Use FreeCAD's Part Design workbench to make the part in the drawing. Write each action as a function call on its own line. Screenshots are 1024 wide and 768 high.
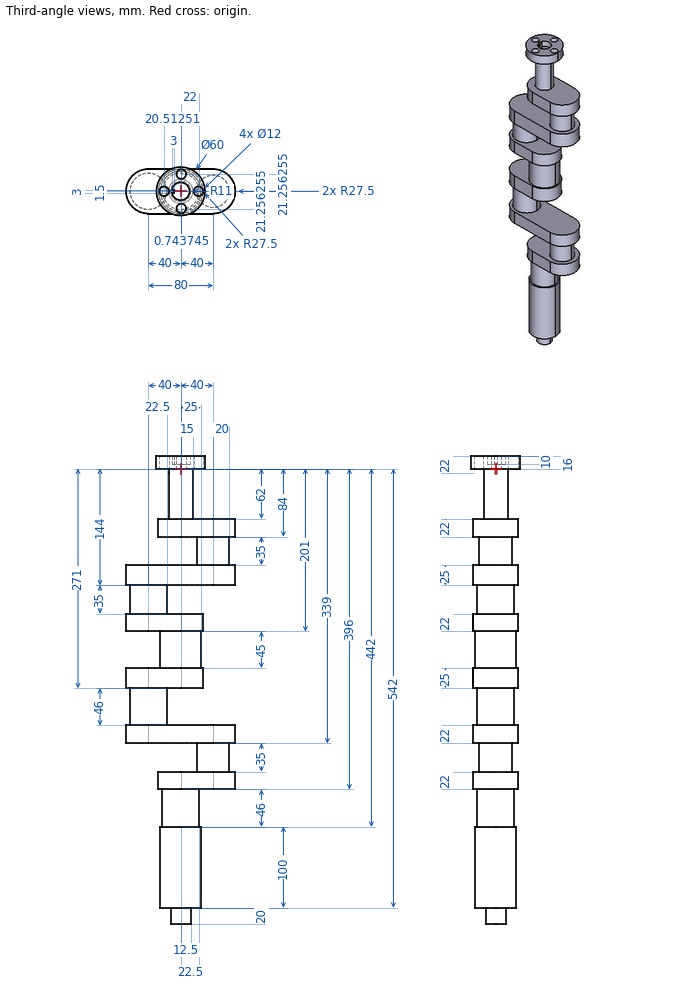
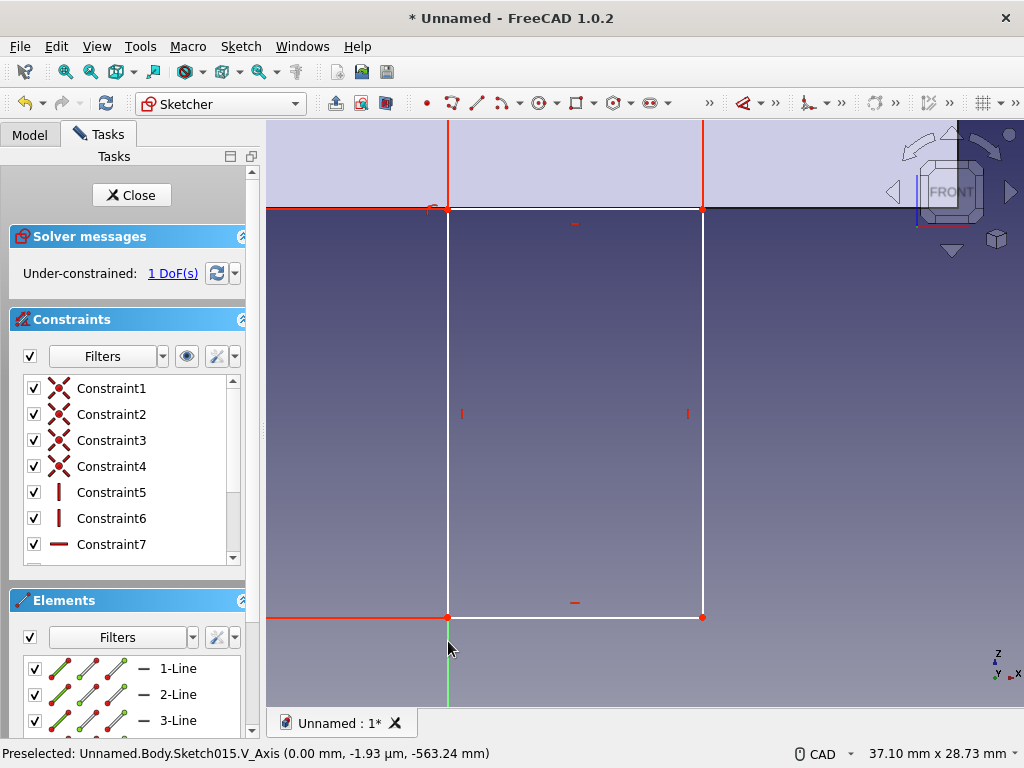
key(d)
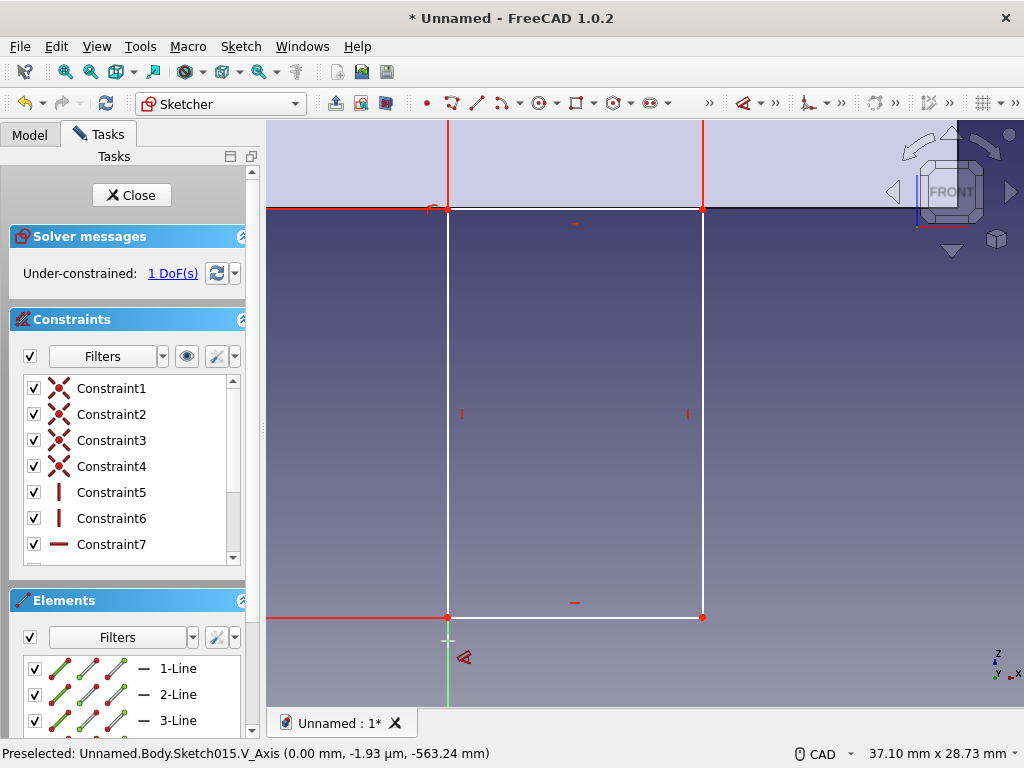
click(448, 209)
click(414, 178)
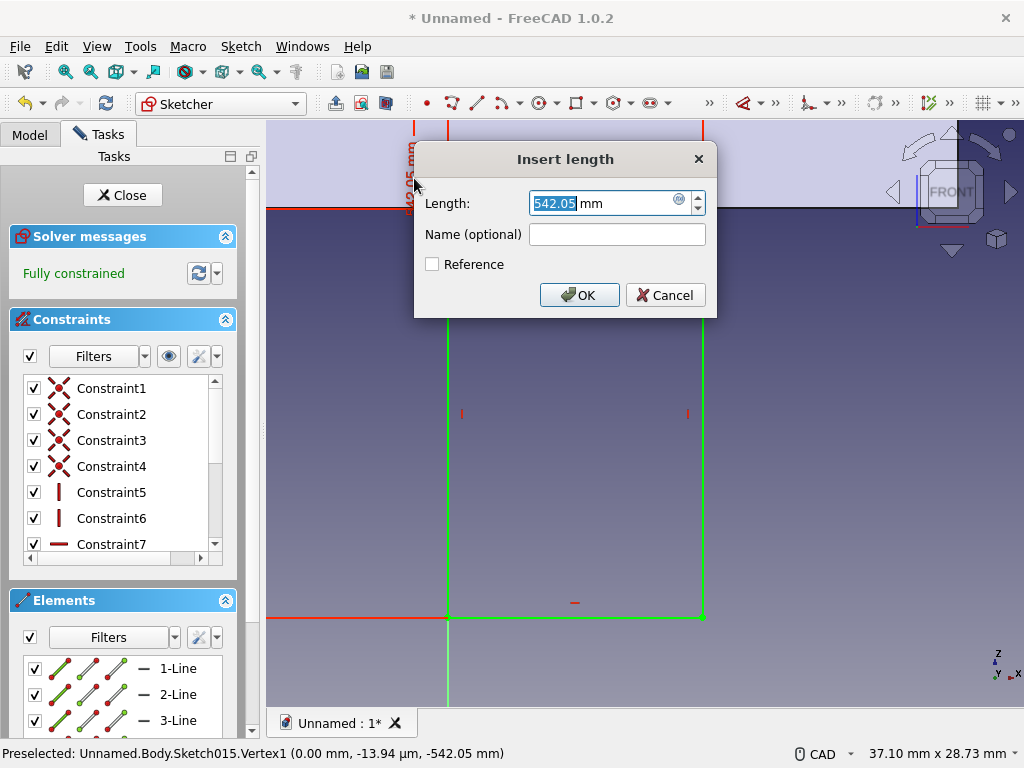
text(542)
key(Return)
key(Escape)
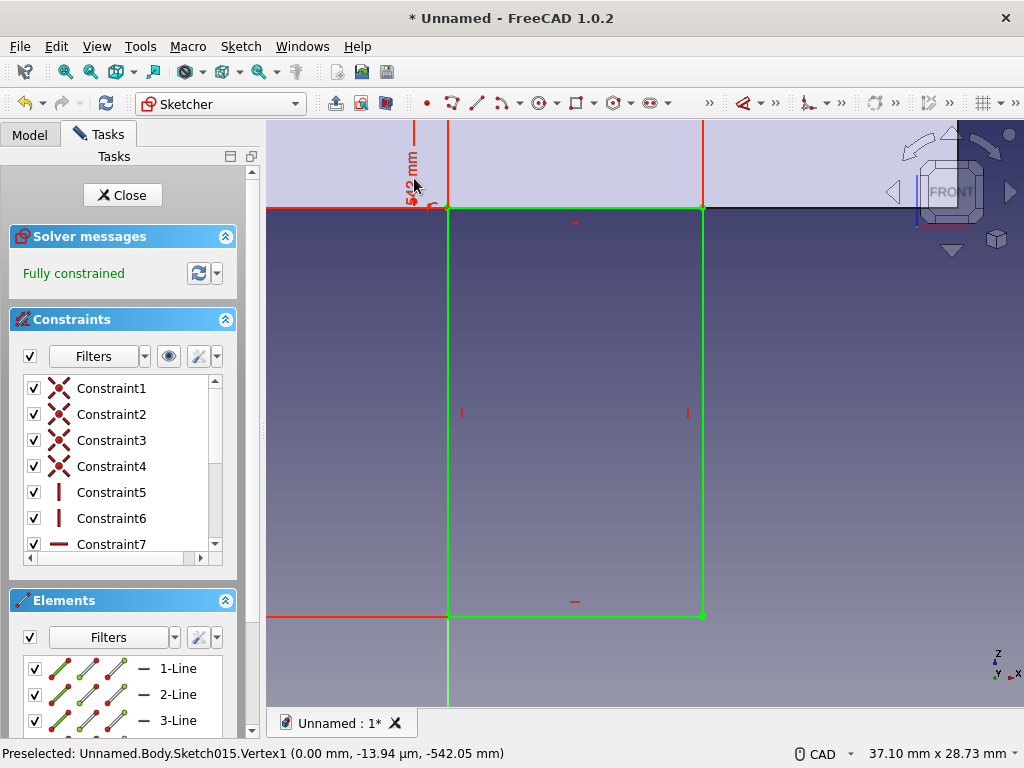
click(123, 195)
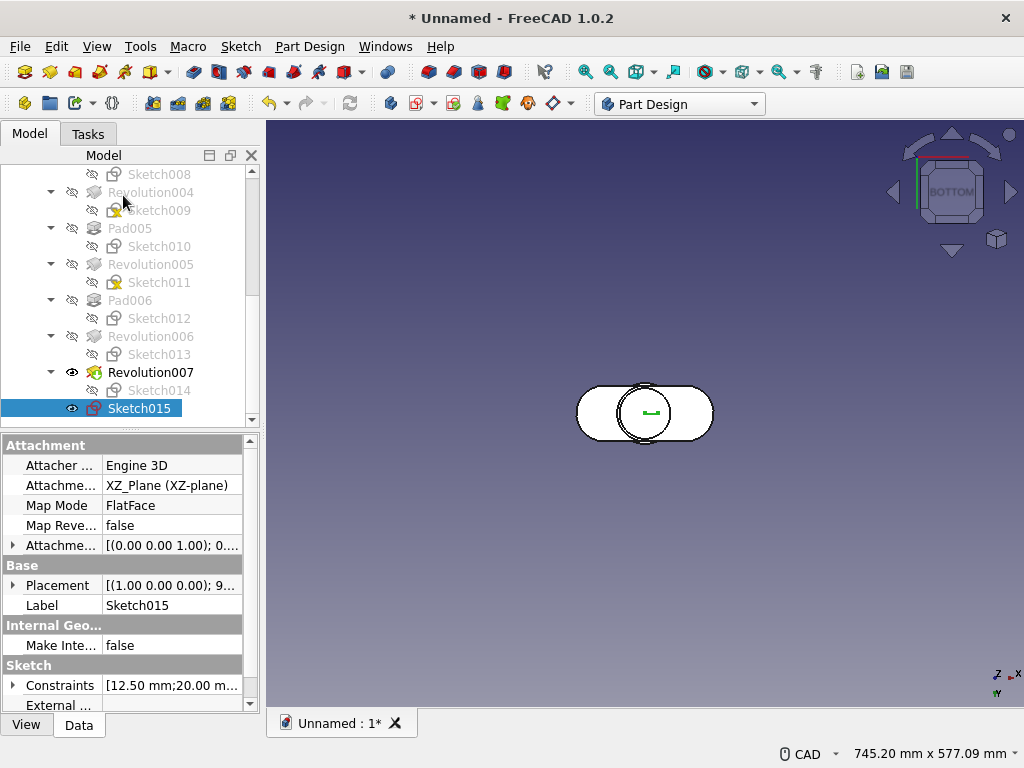
click(50, 72)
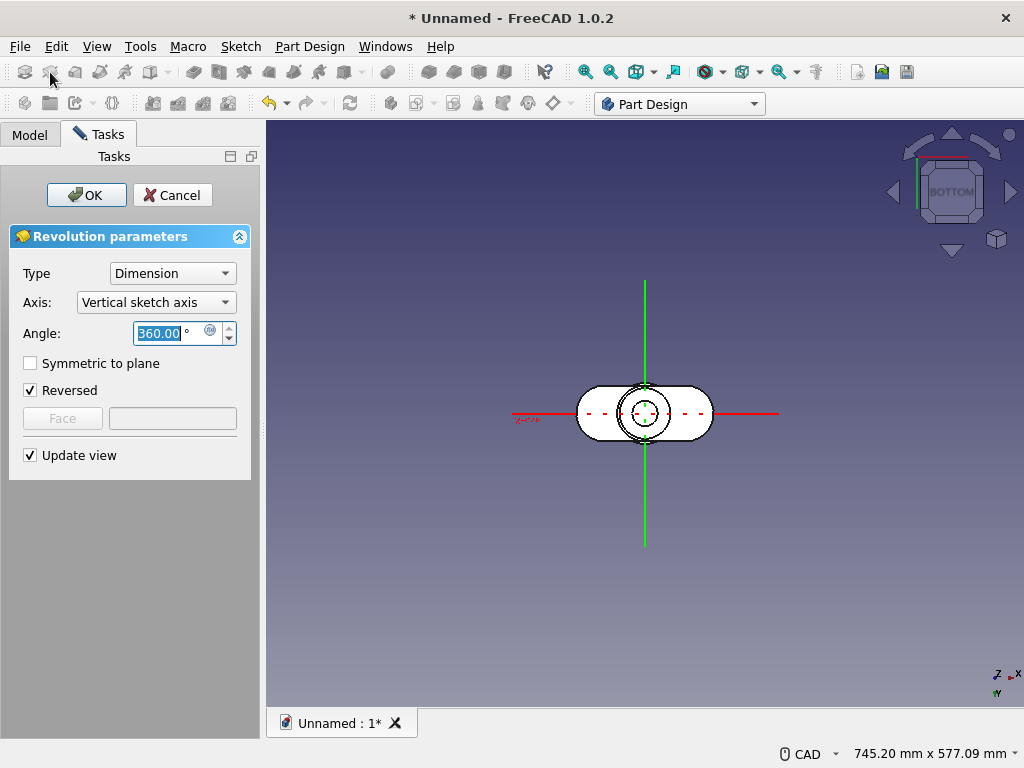
click(87, 195)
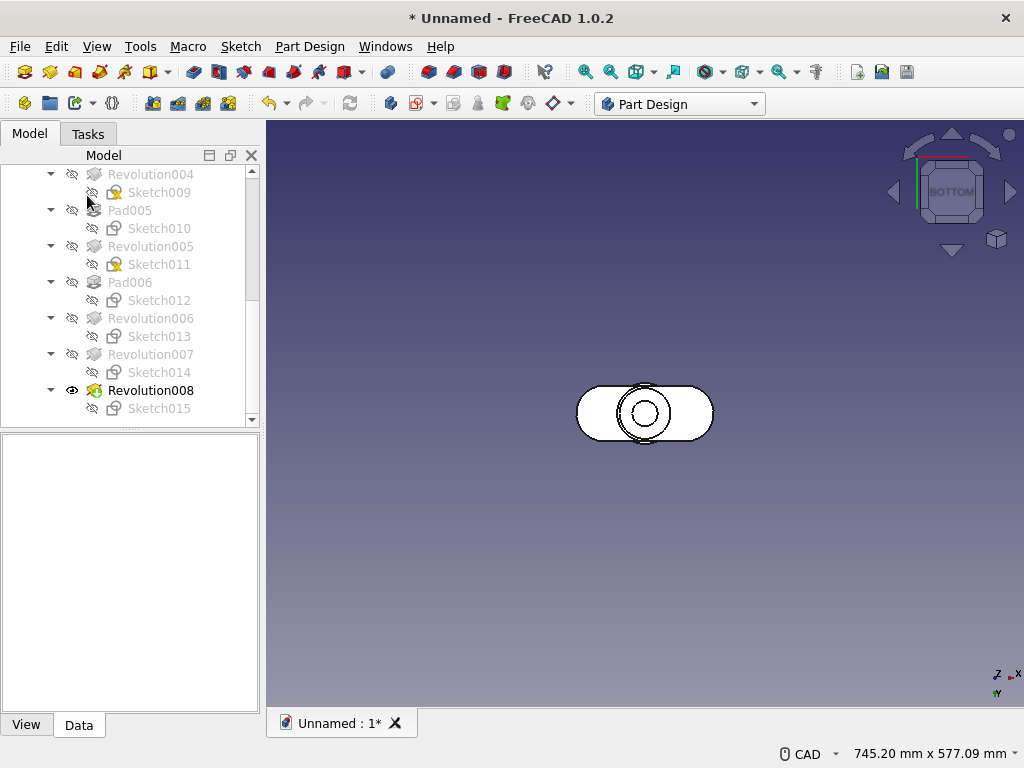
key(v)
key(f)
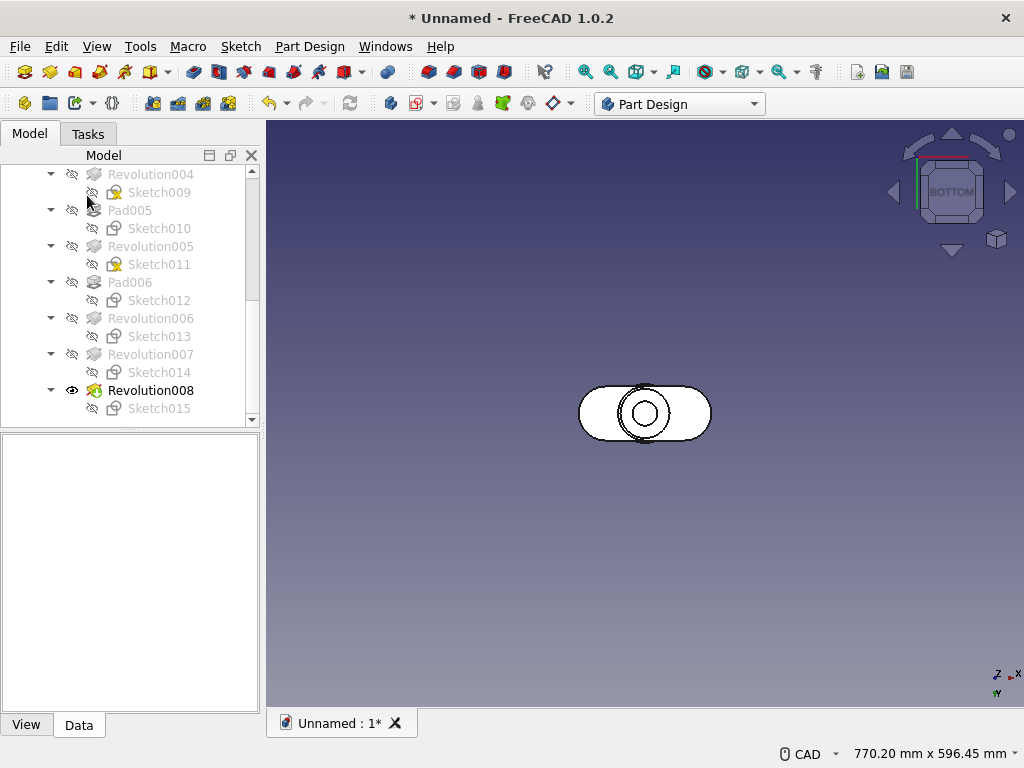
key(0)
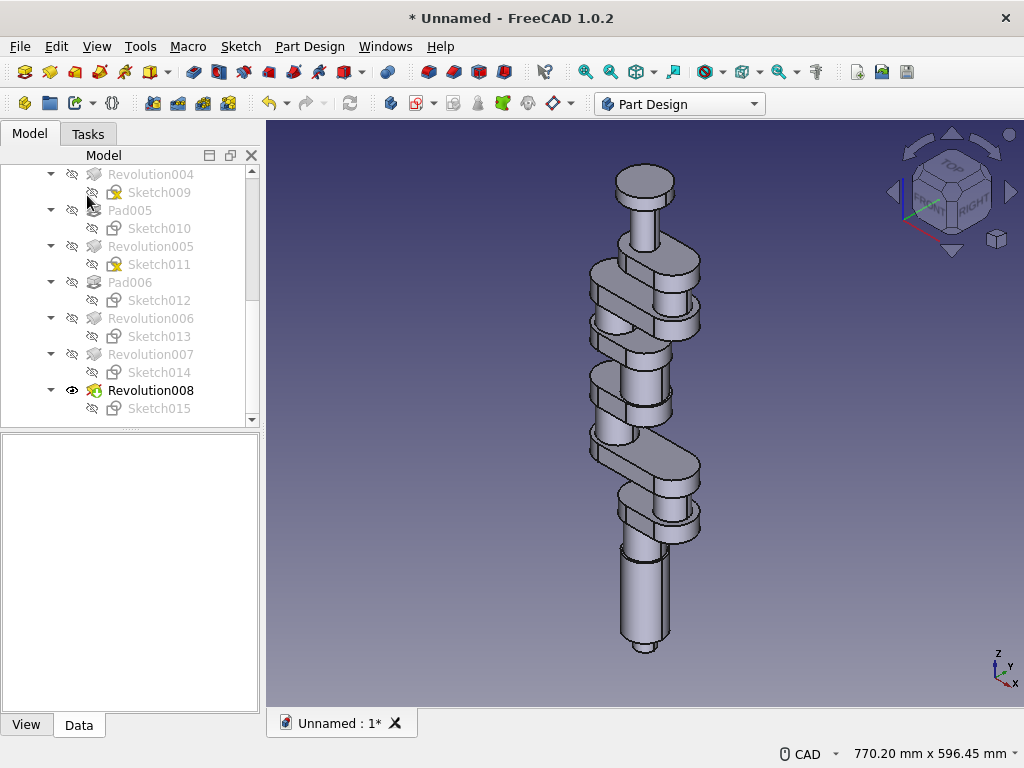
click(645, 180)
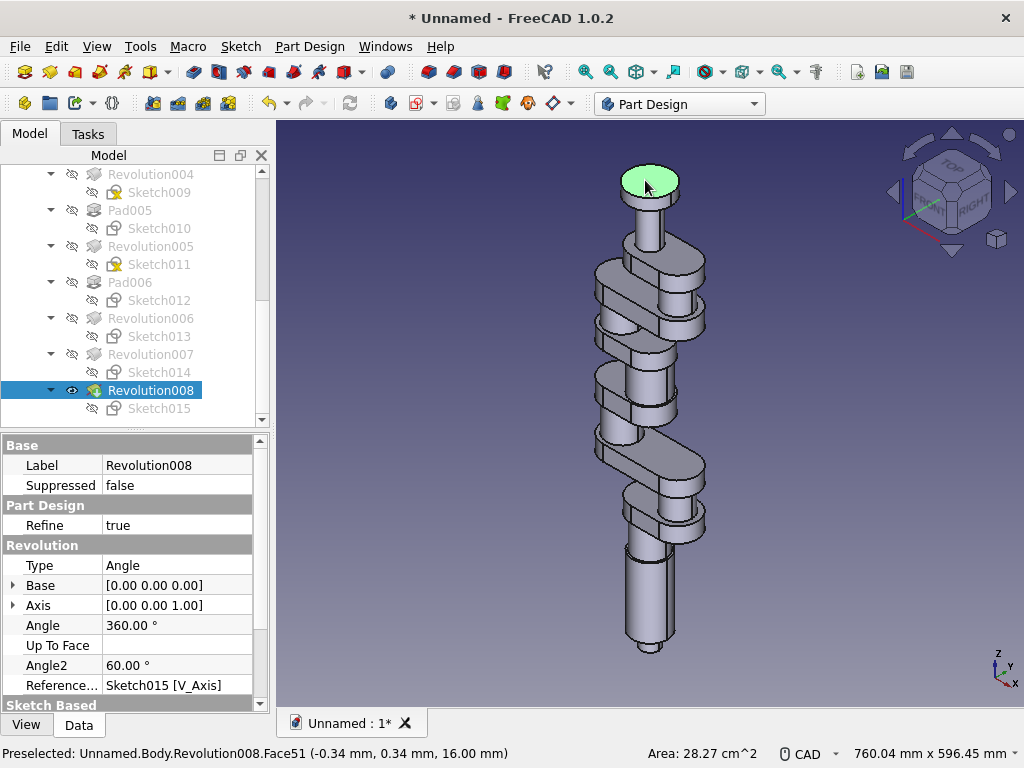
click(416, 104)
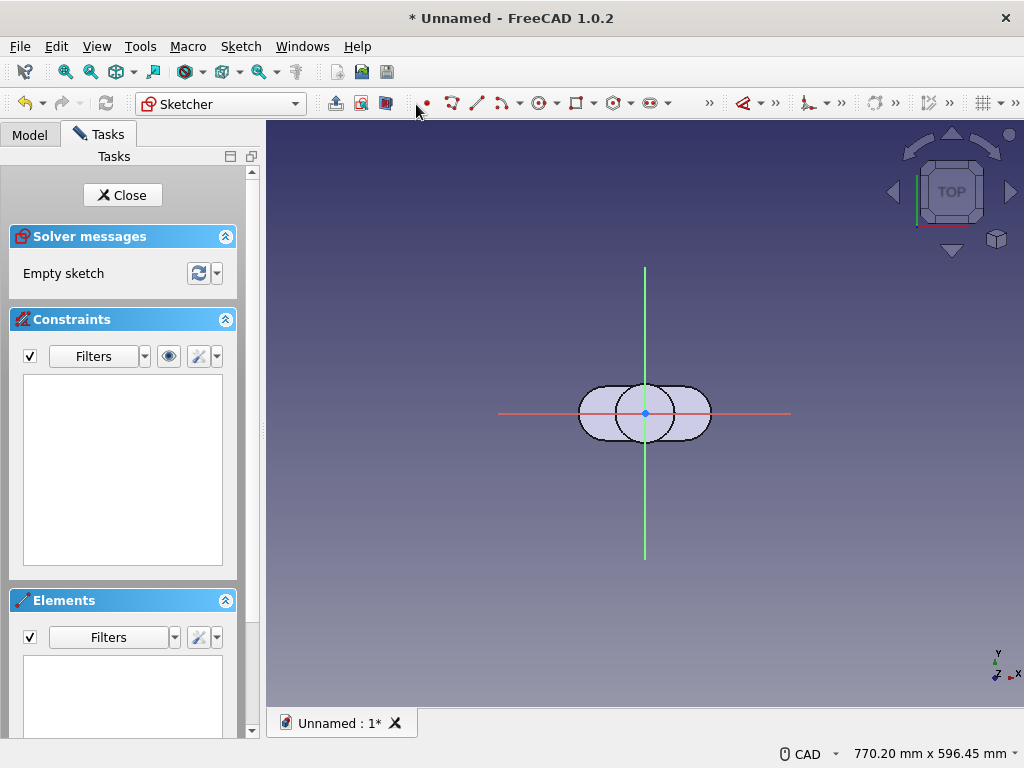
scroll(657, 414, up, 10)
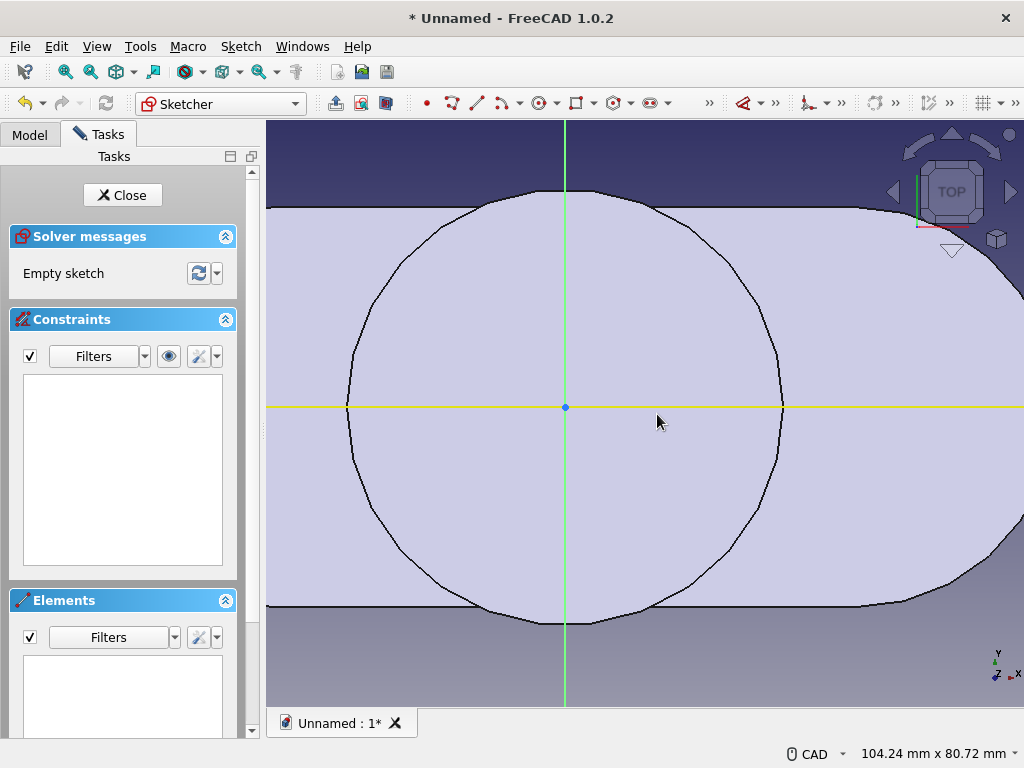
key(g)
key(c)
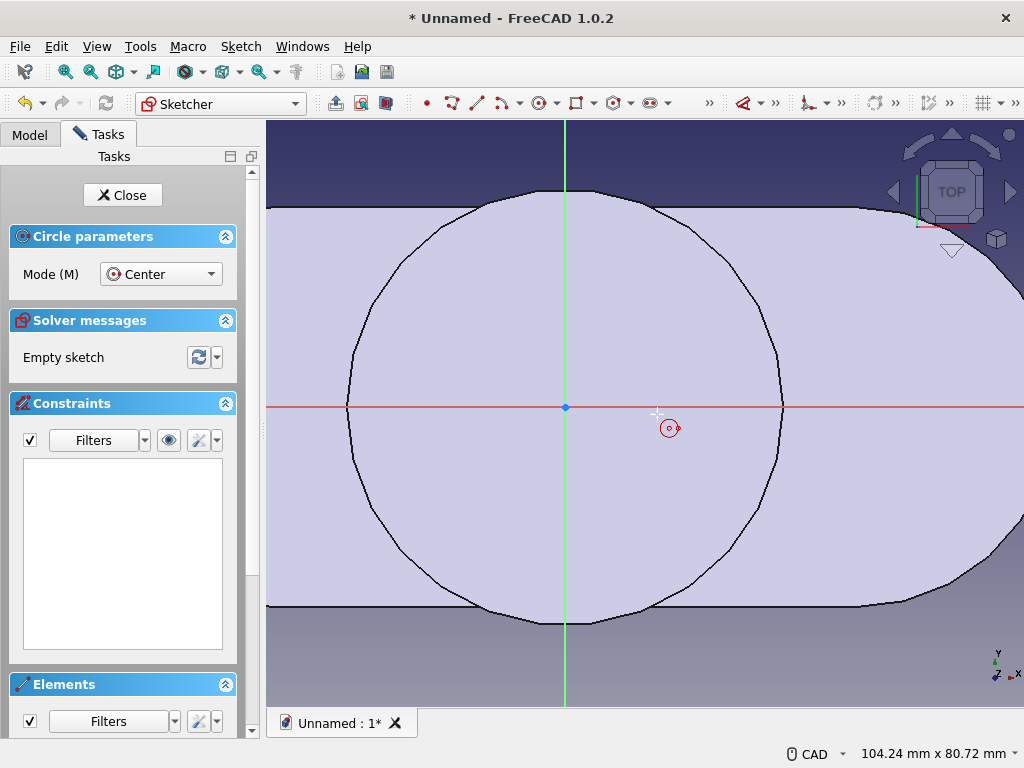
click(725, 407)
move(756, 376)